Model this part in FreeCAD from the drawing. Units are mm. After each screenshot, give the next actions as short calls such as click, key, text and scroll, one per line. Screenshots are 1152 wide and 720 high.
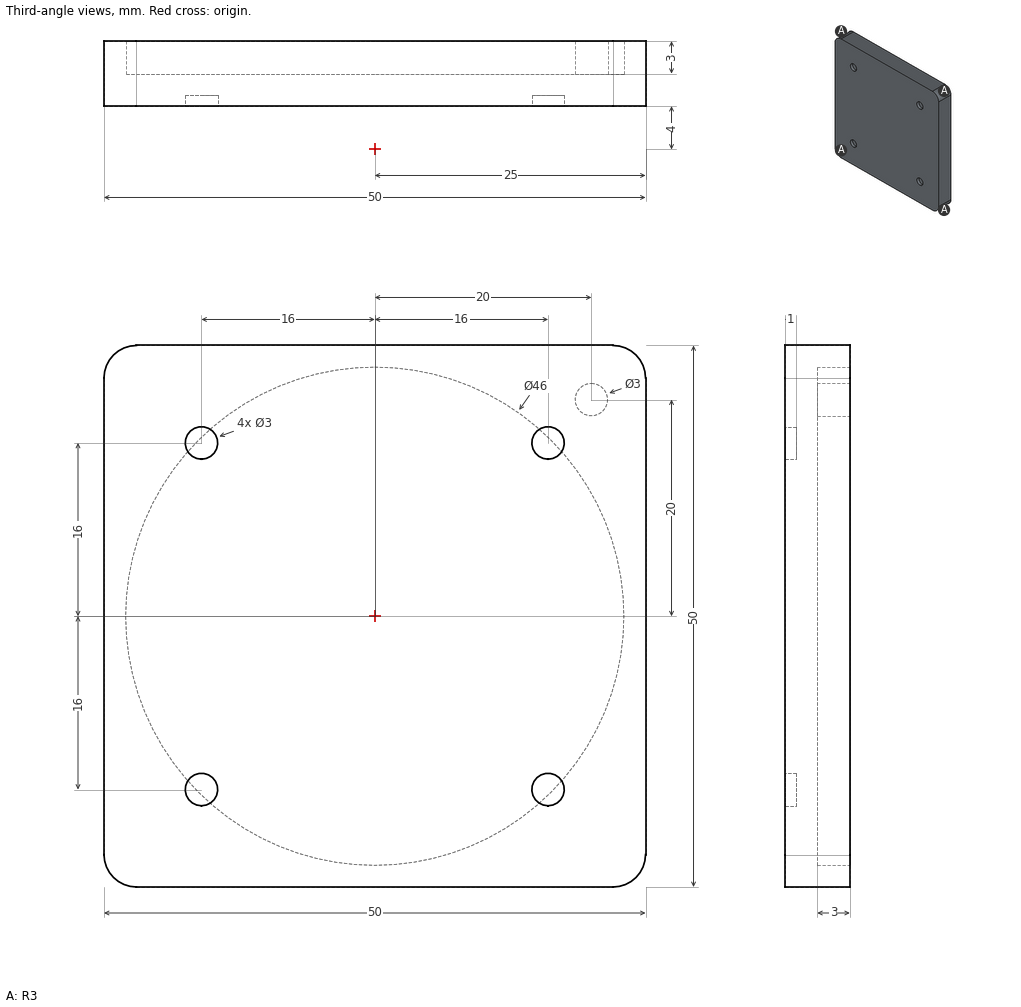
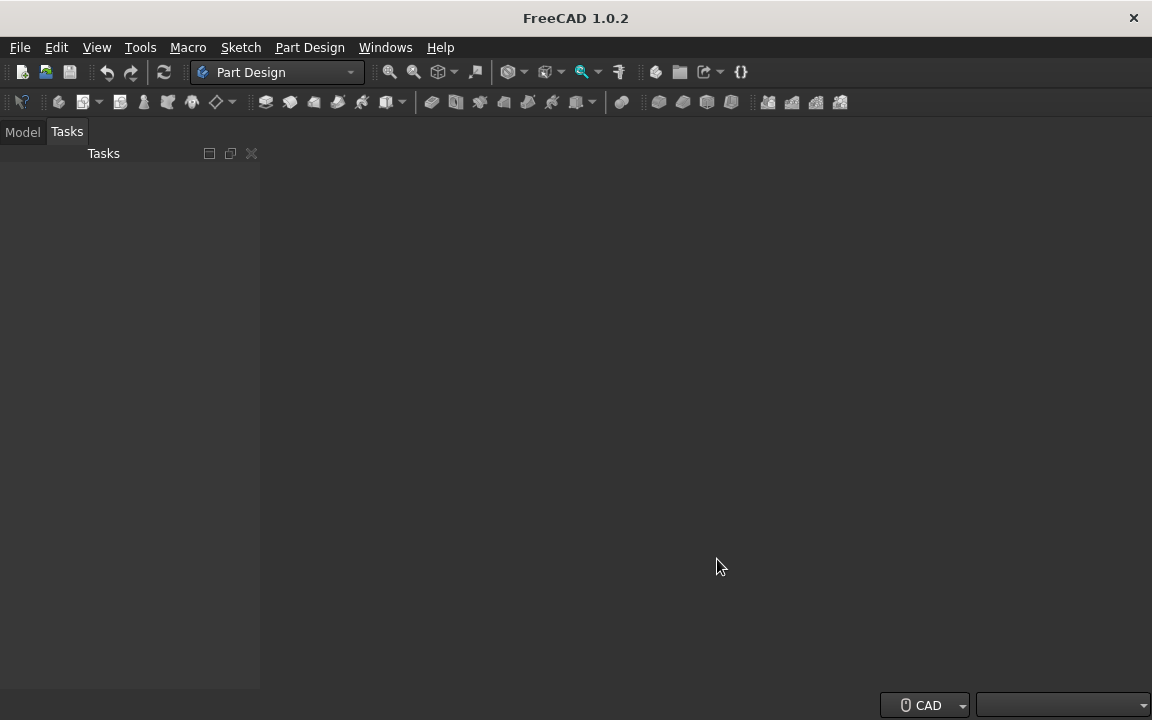
key(ctrl+n)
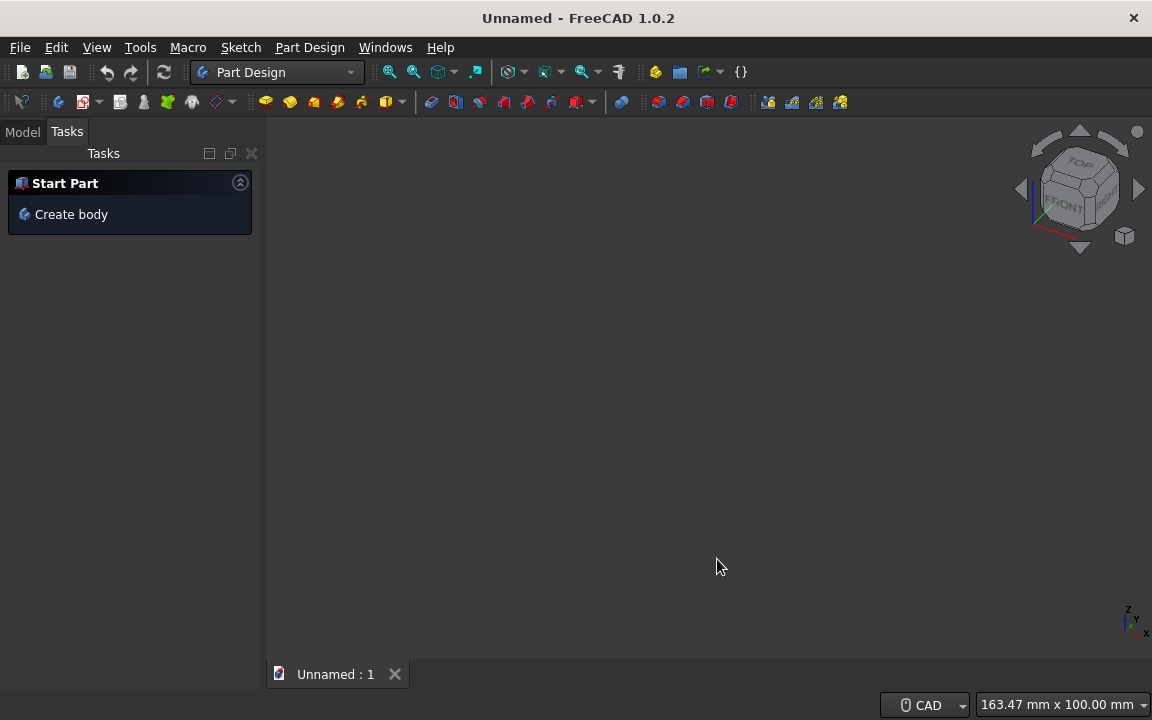
click(84, 102)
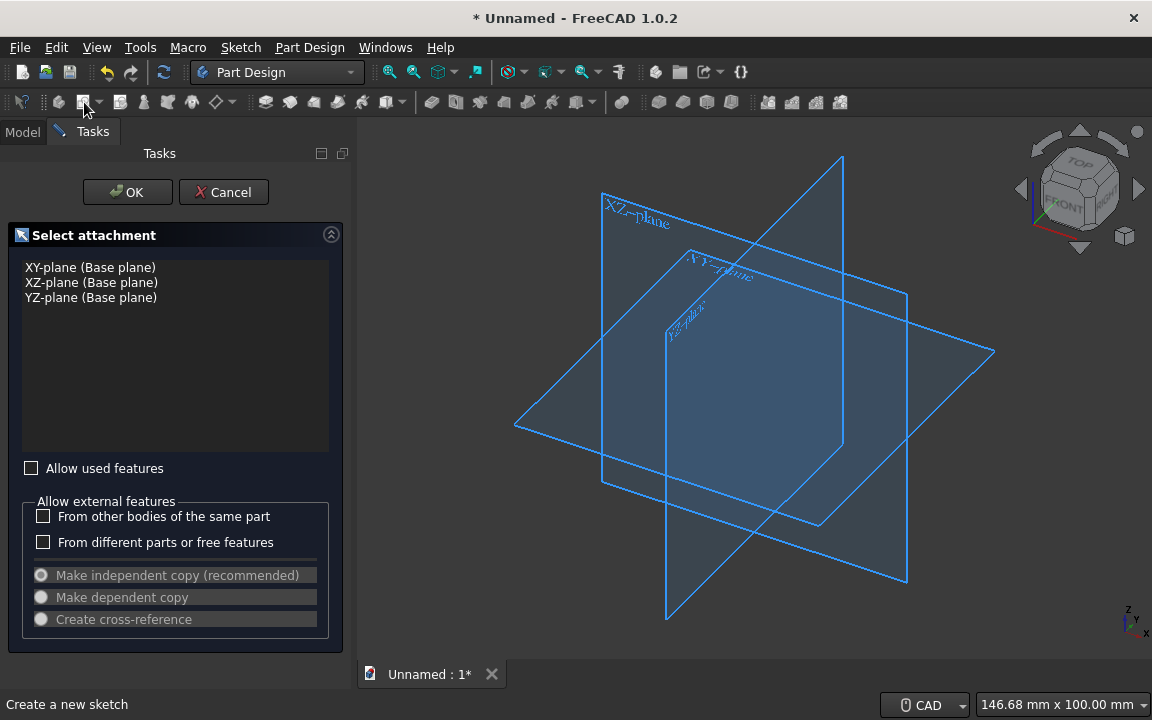
click(82, 282)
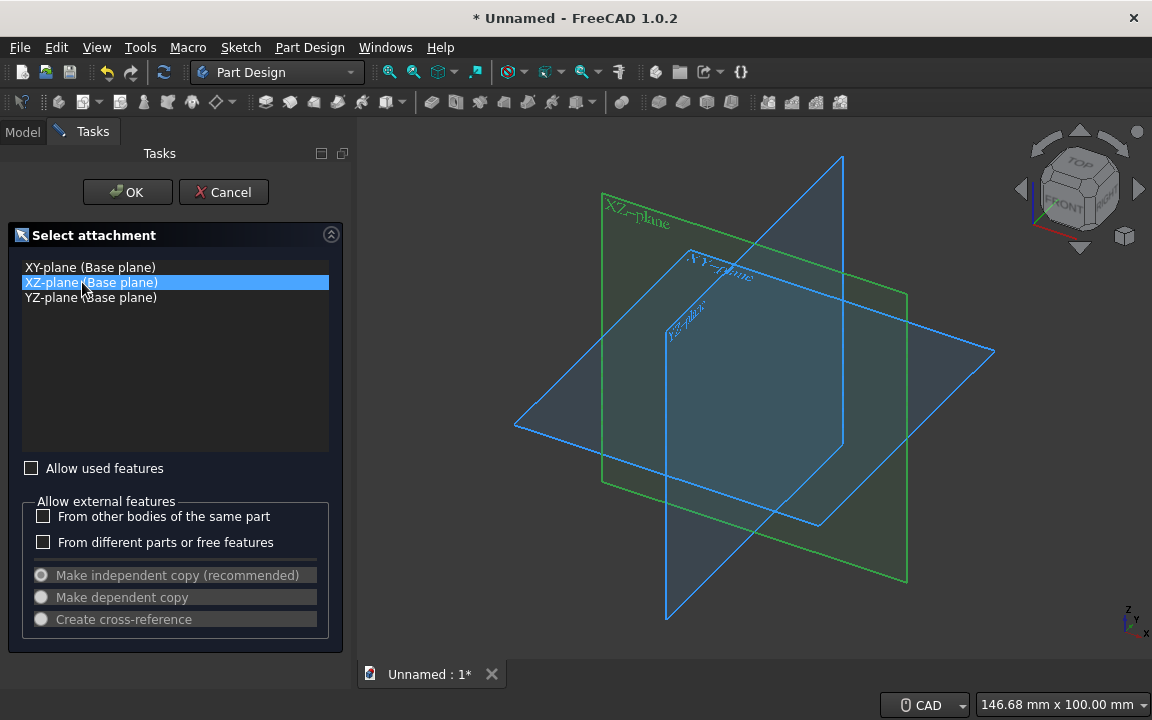
click(128, 192)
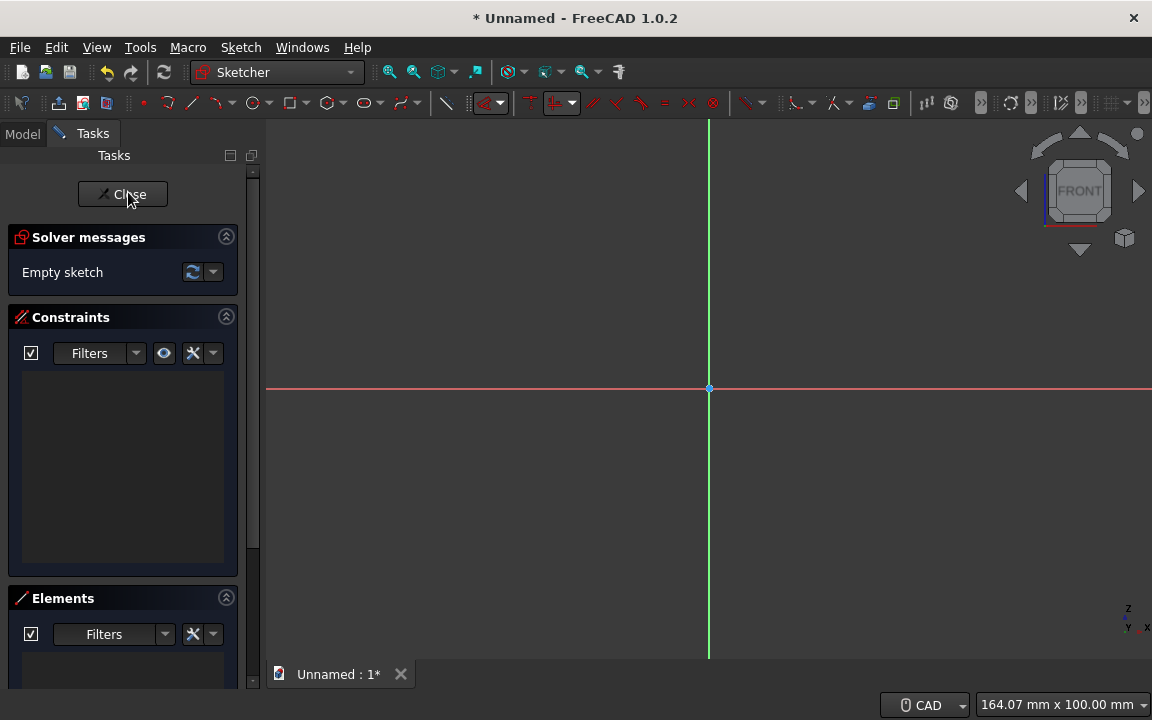
key(g)
key(v)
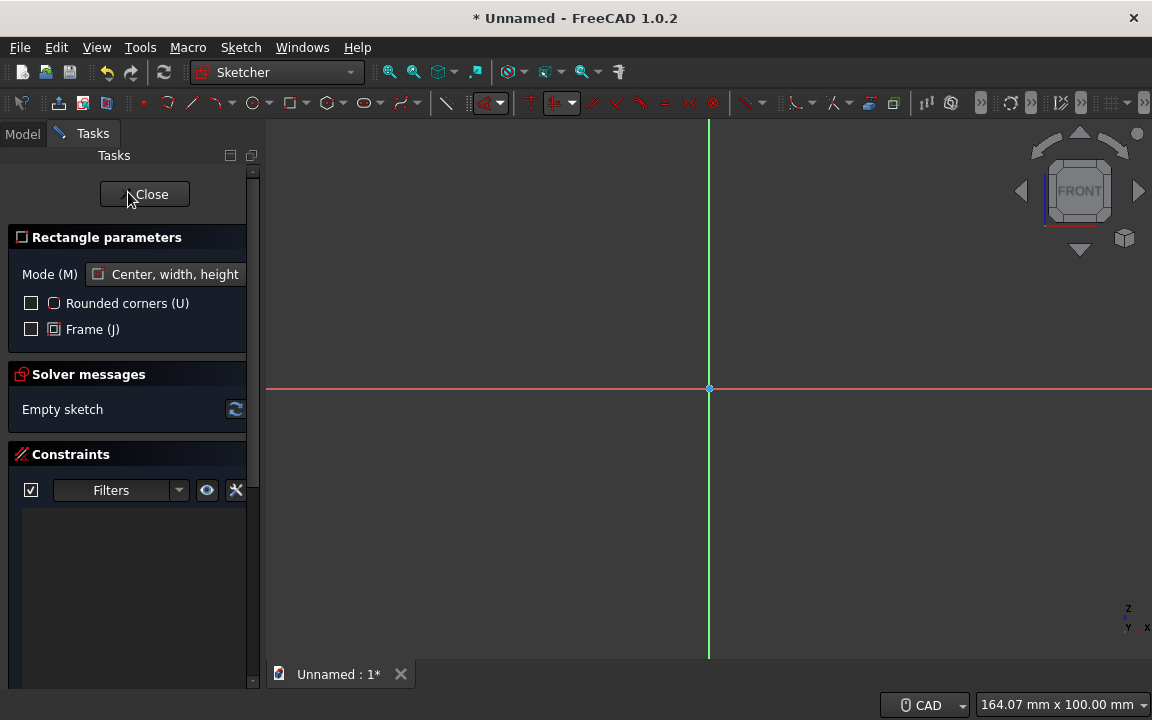
click(709, 389)
click(844, 254)
key(Escape)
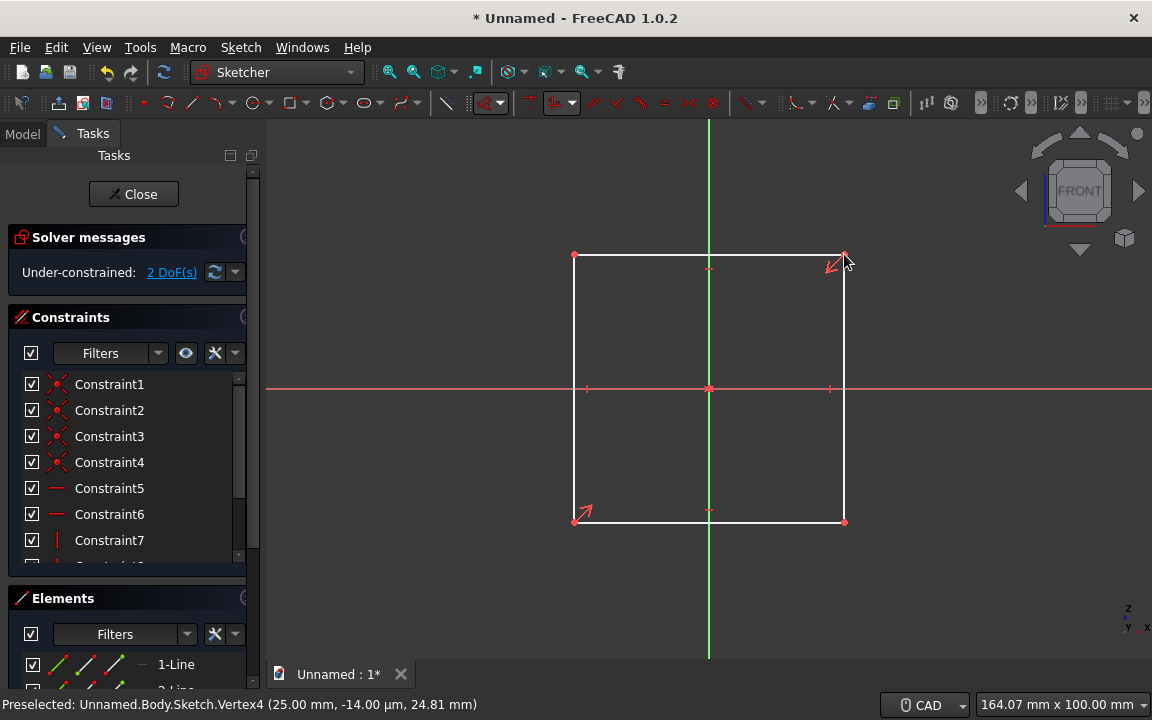
click(655, 523)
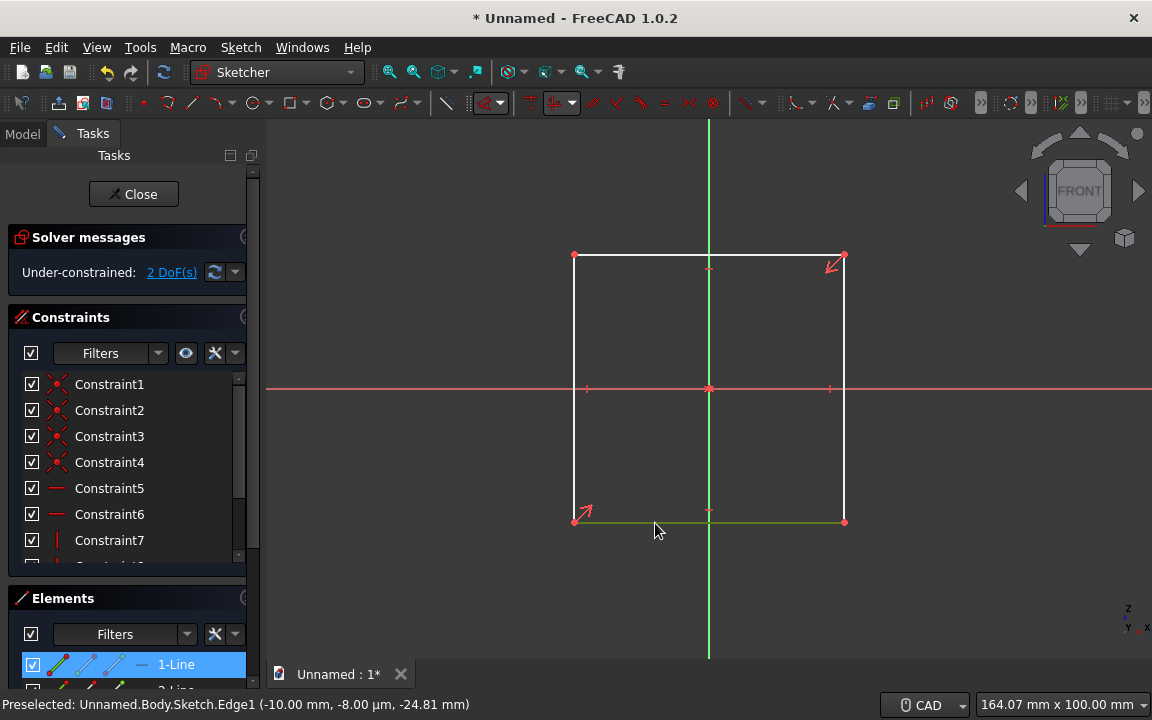
click(502, 104)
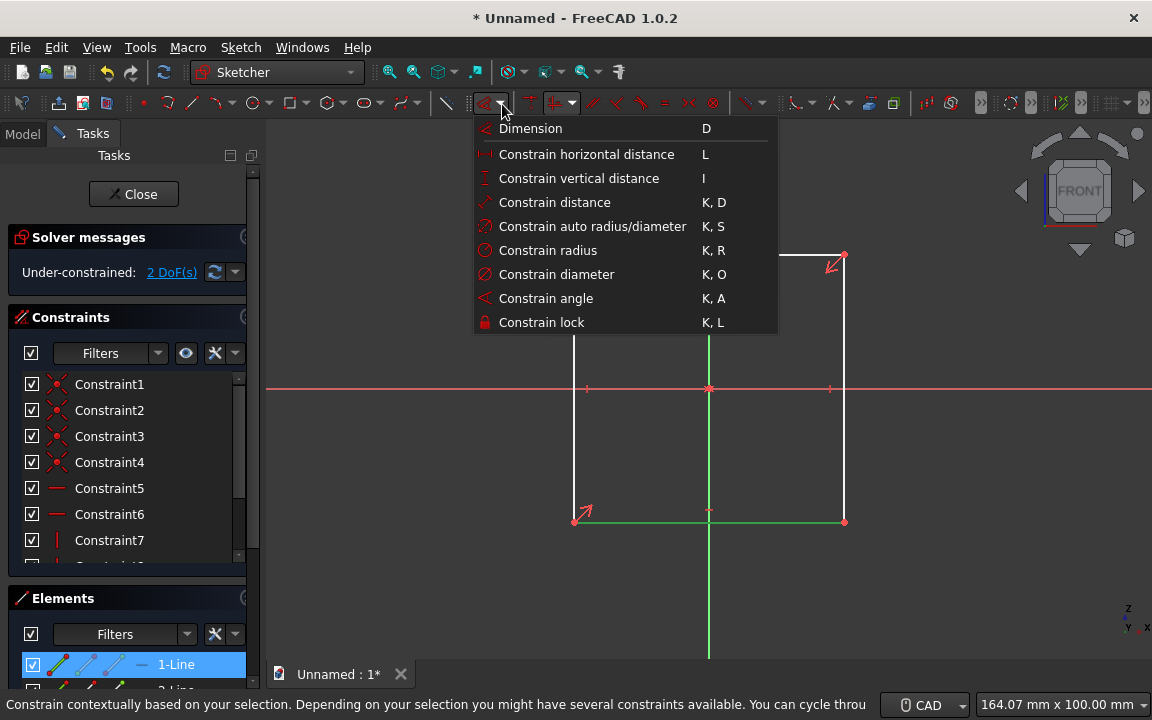
click(626, 154)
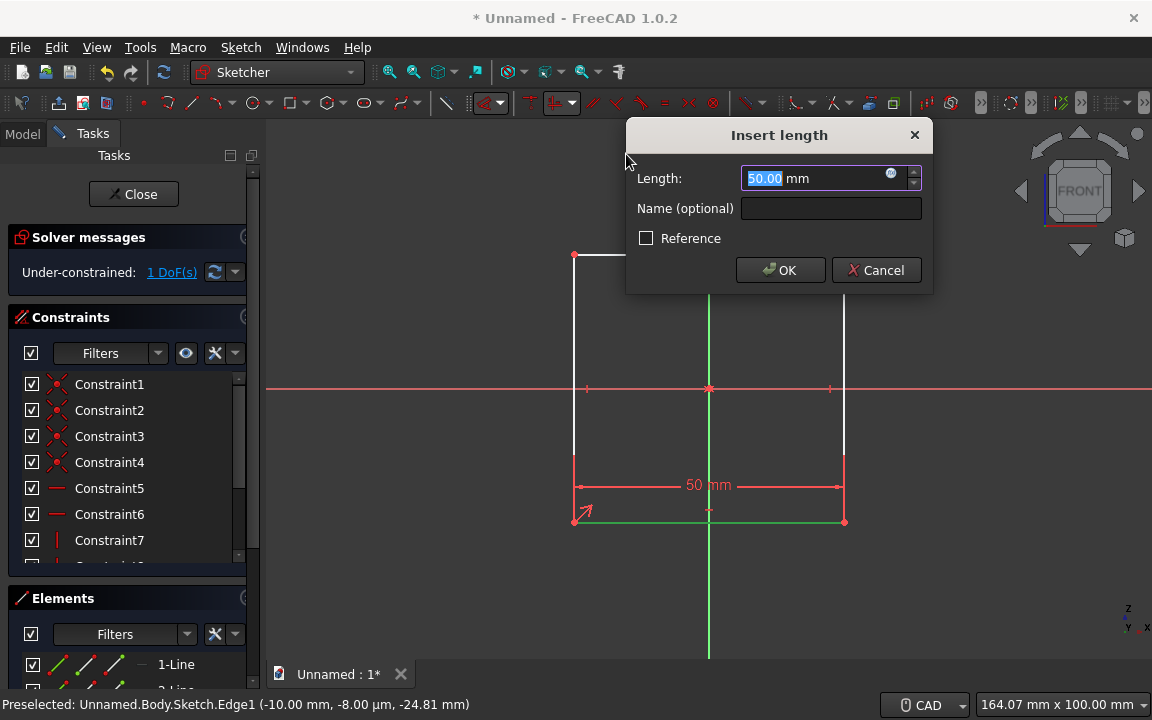
text(50)
key(Return)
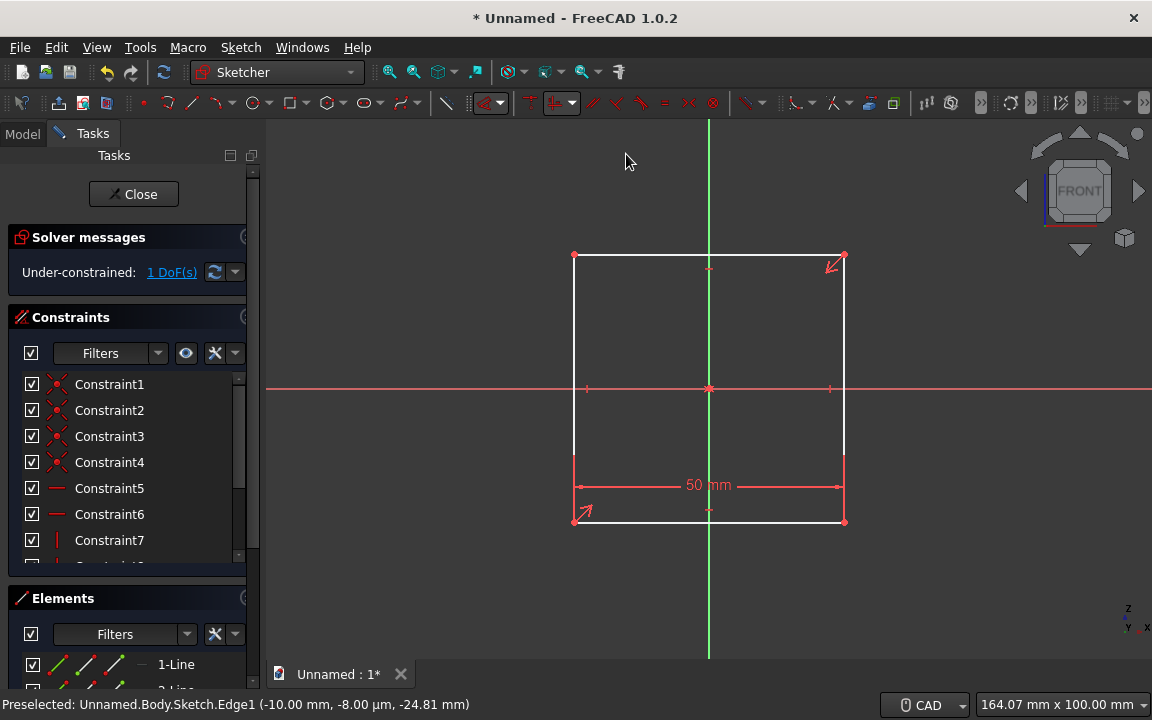
click(844, 443)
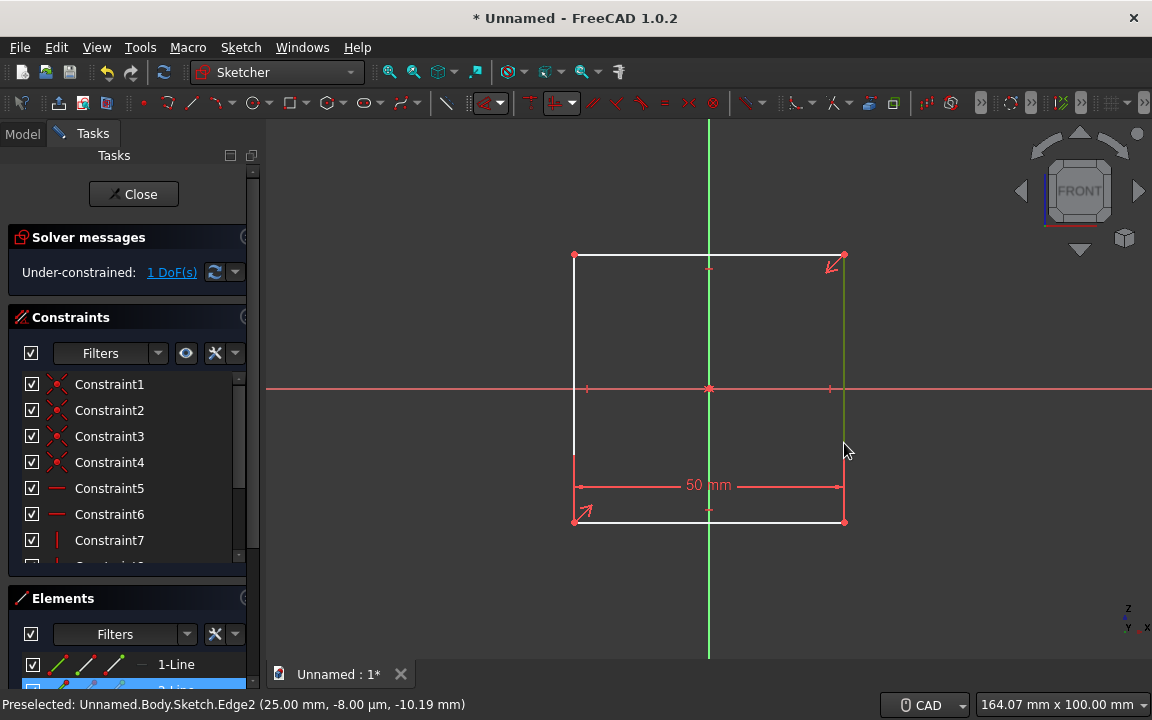
key(i)